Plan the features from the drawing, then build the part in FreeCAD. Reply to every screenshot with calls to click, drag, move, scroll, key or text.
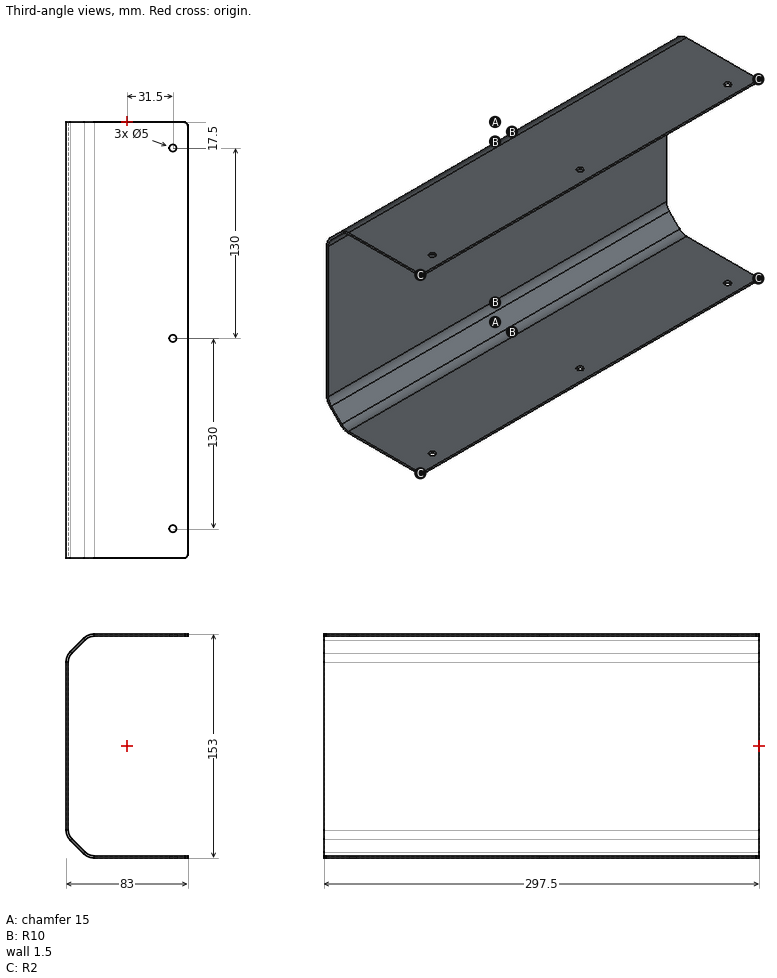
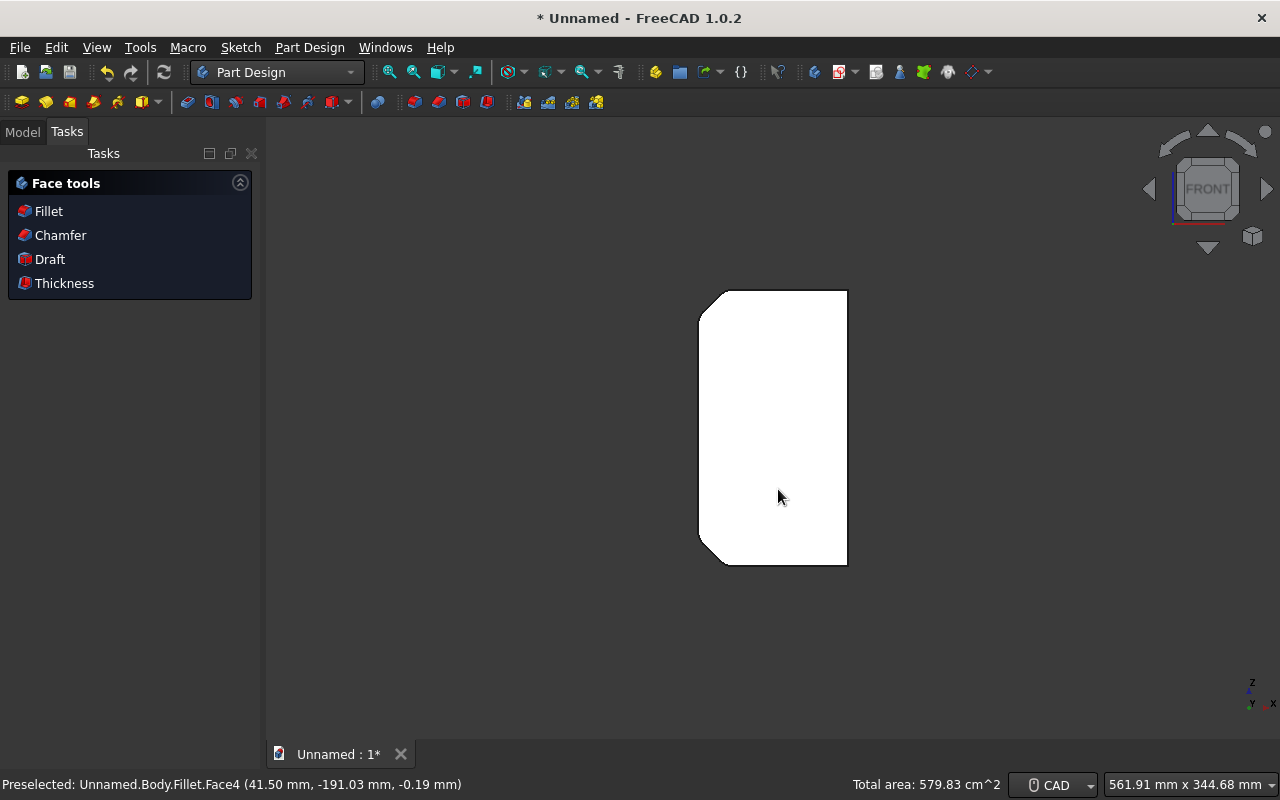
key(3)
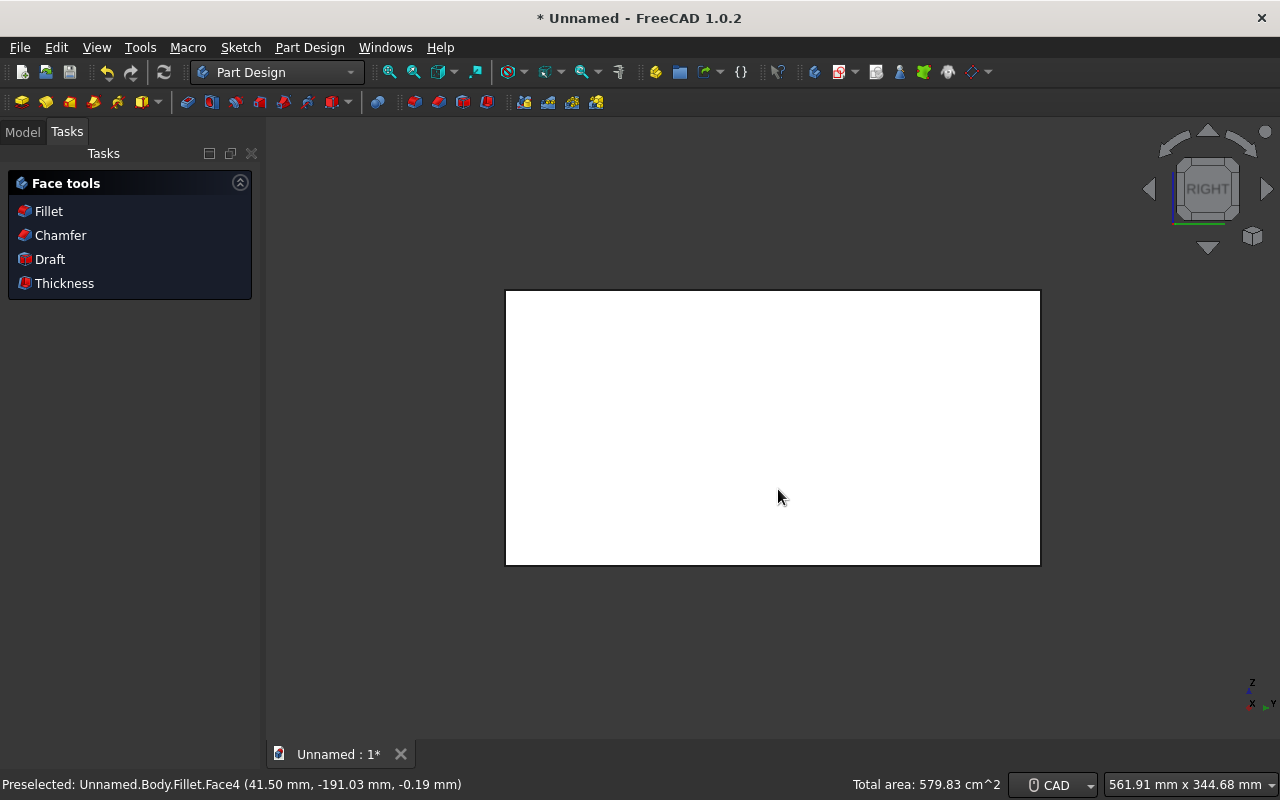
key(5)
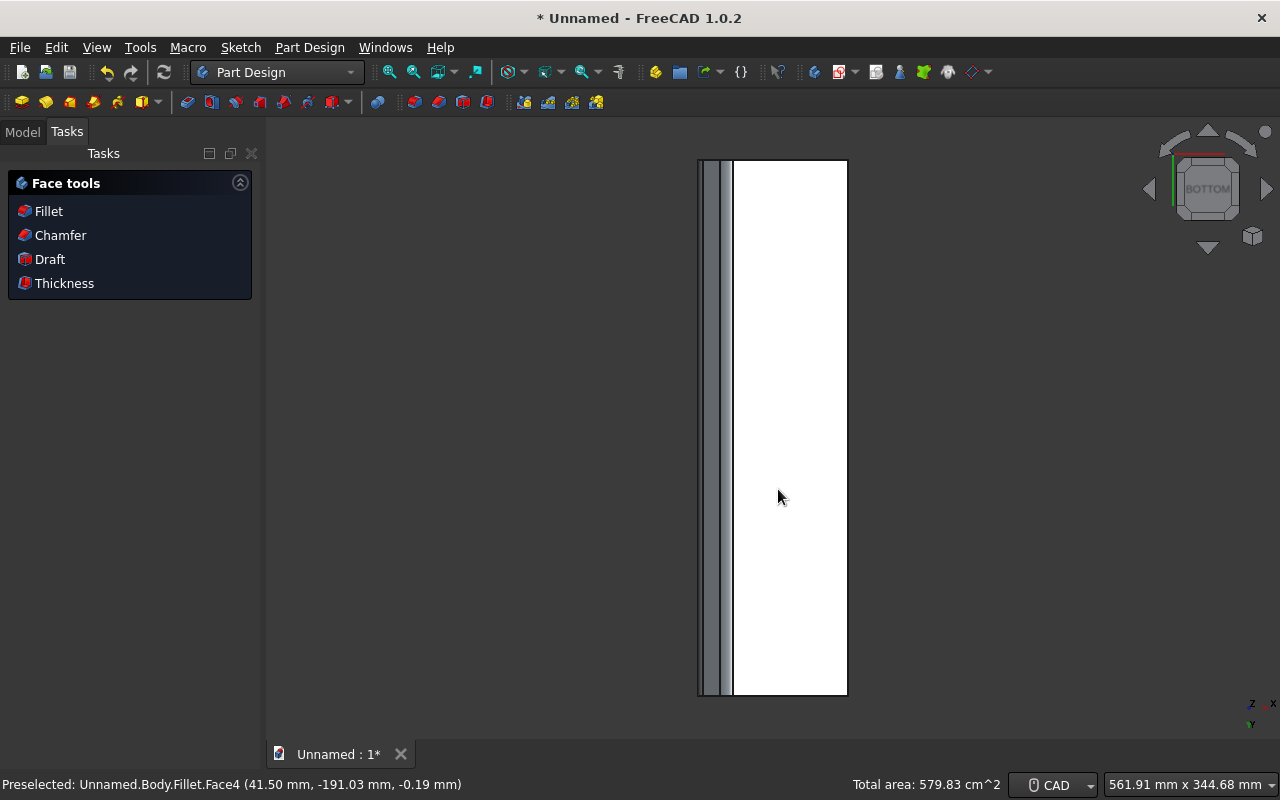
key(4)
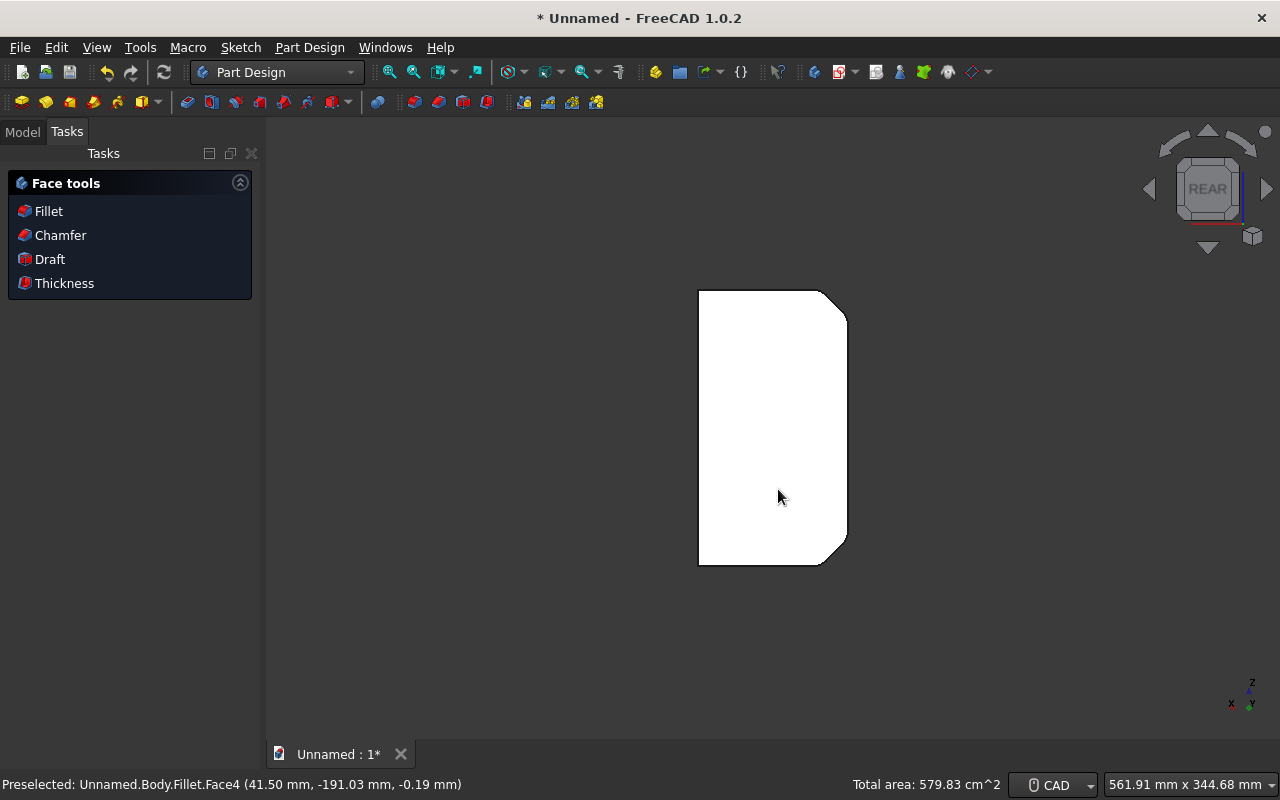
key(v)
key(f)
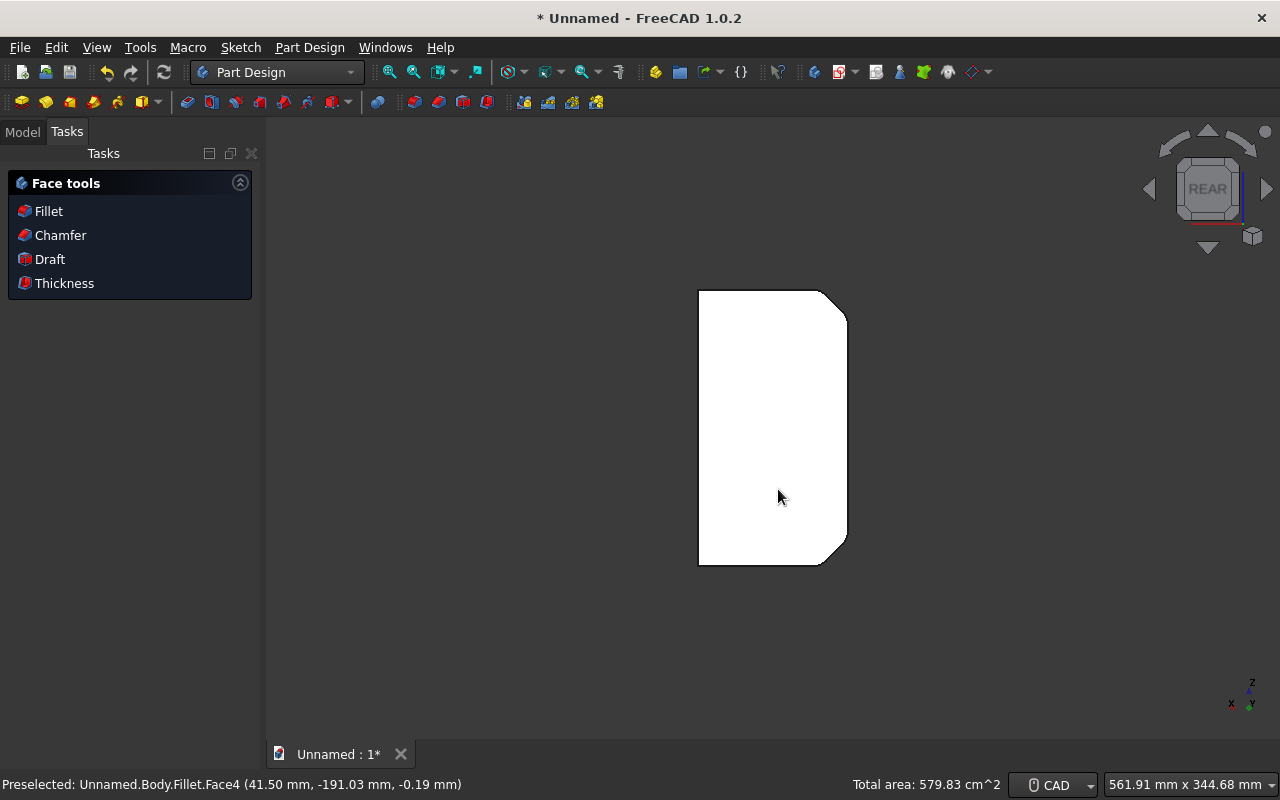
click(773, 388, ctrl)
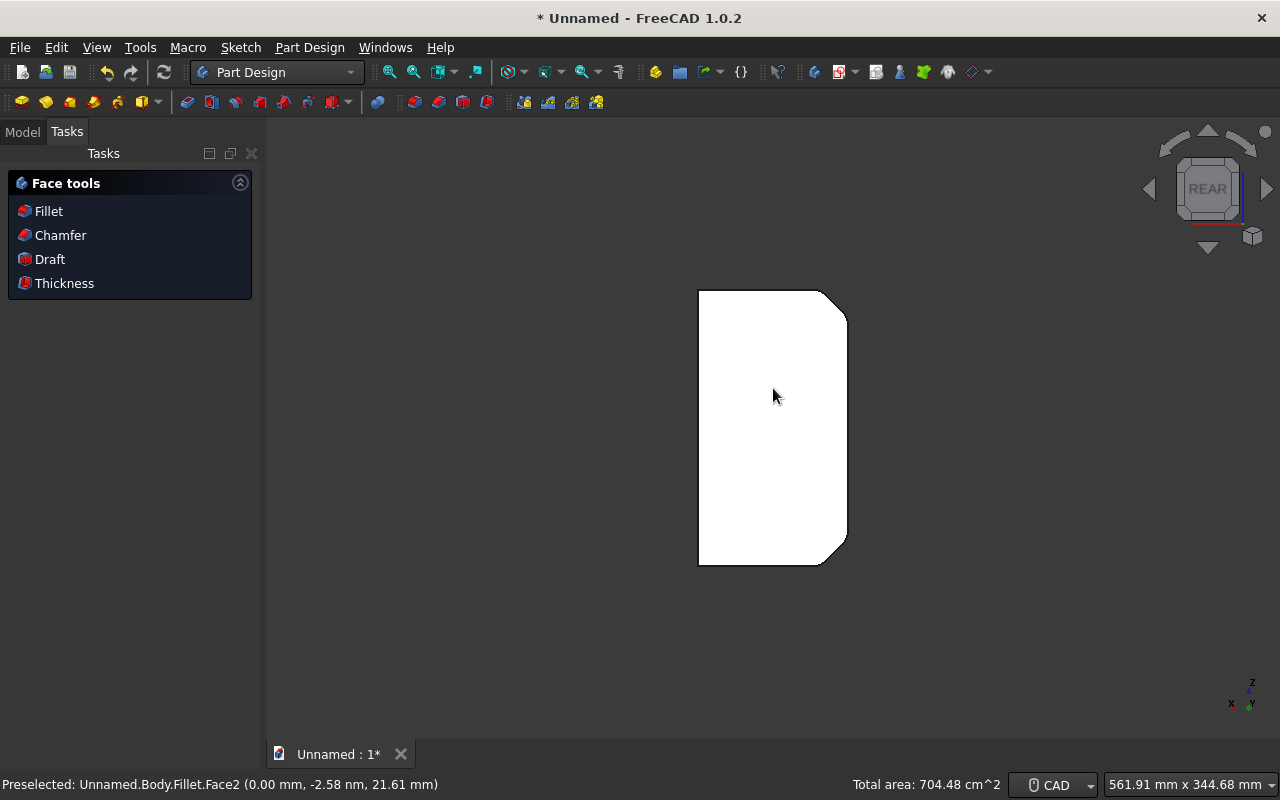
click(488, 102)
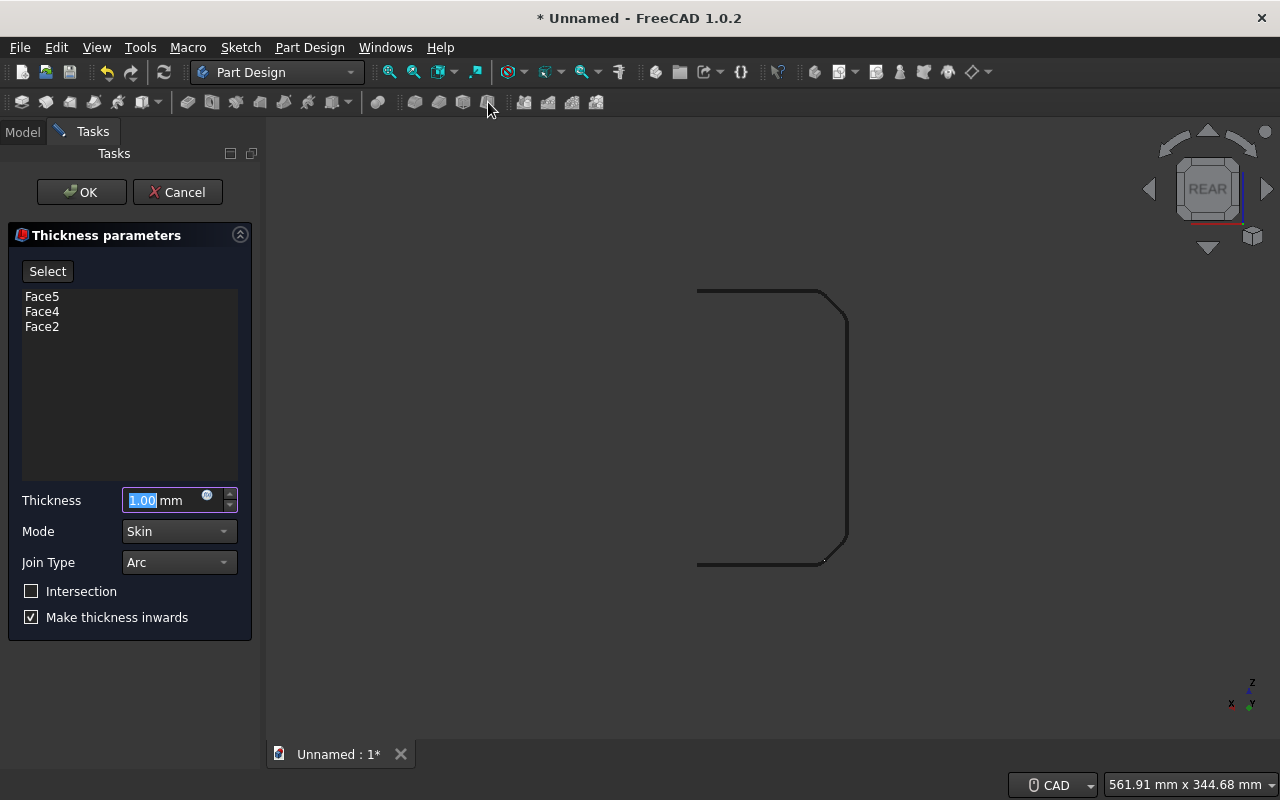
text(1.5)
key(Tab)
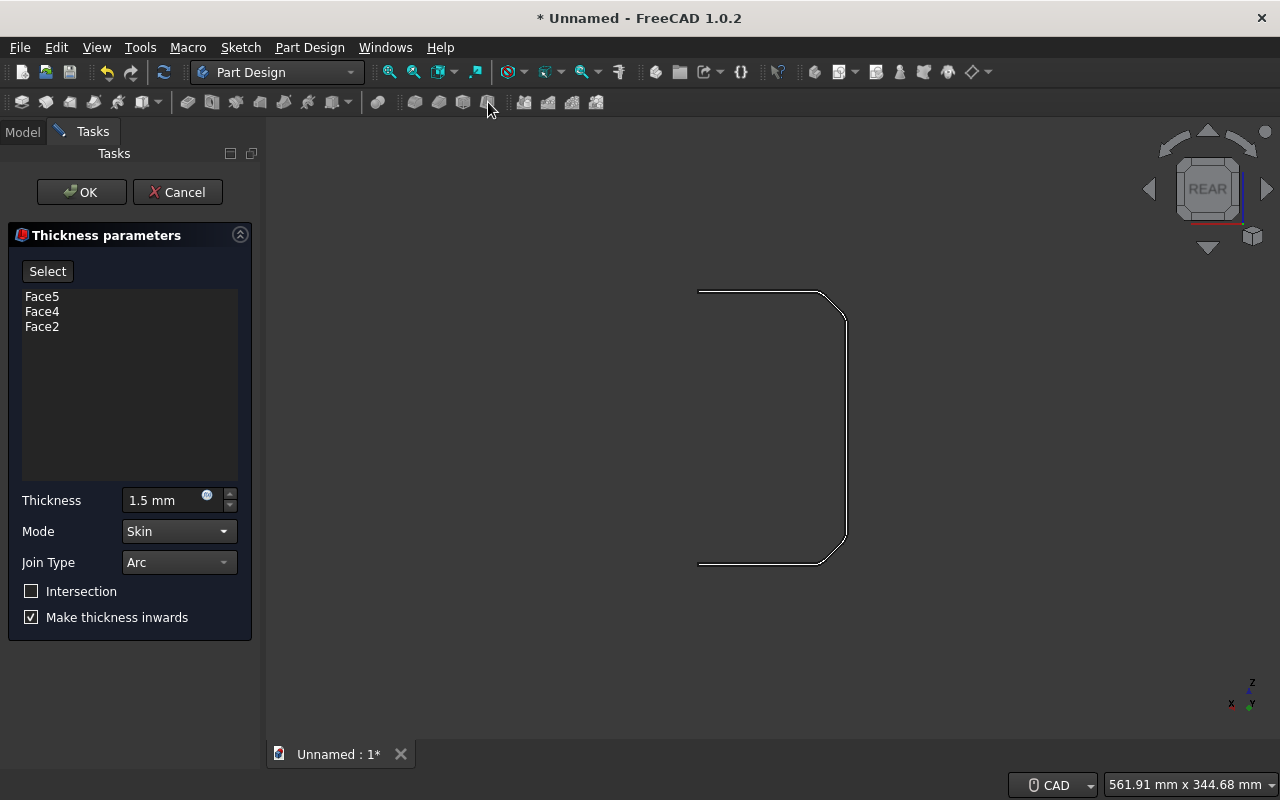
click(180, 562)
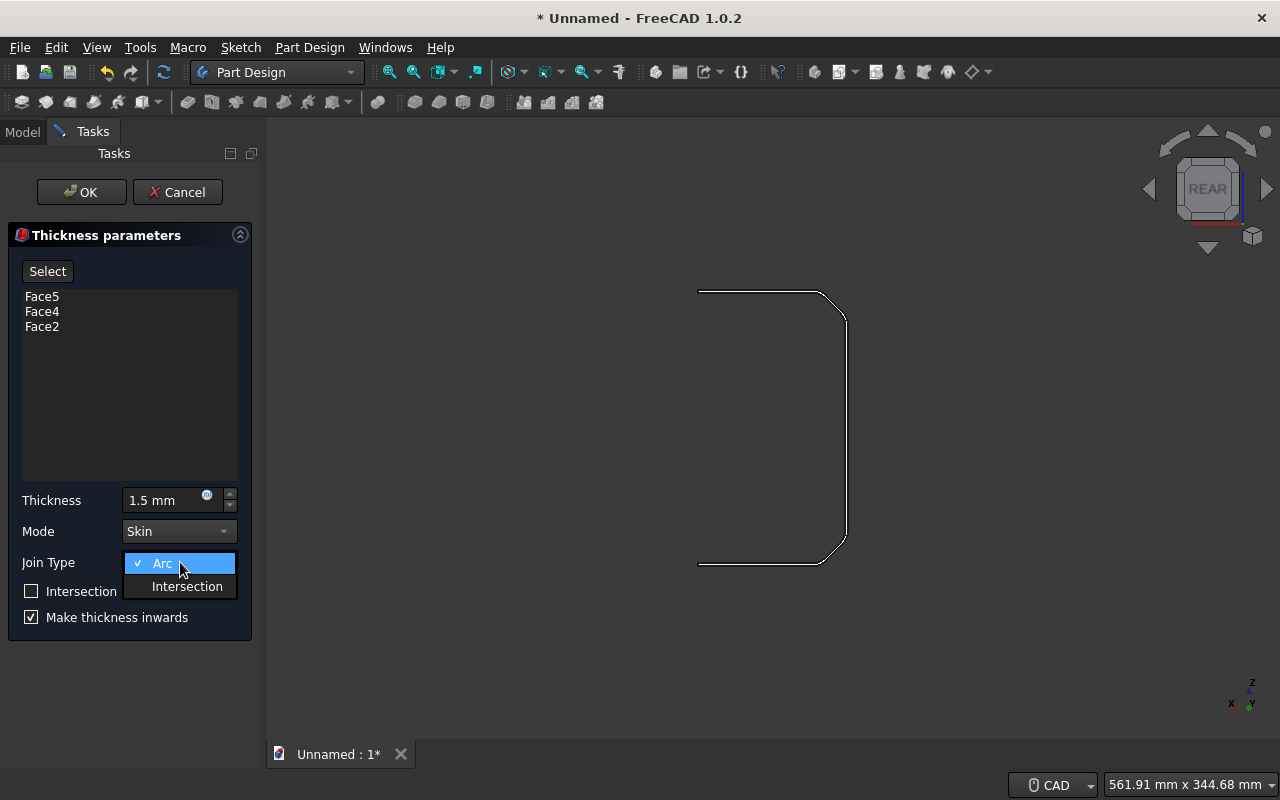
click(179, 586)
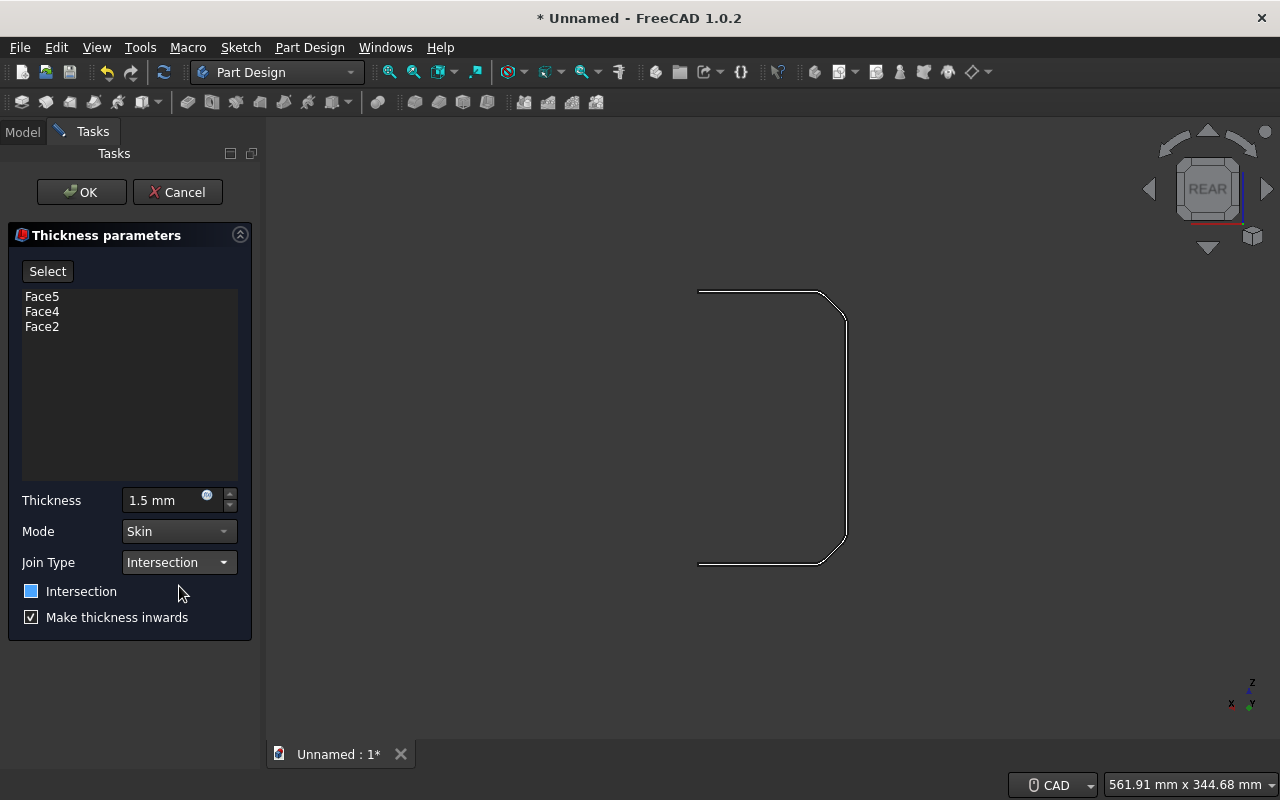
click(82, 192)